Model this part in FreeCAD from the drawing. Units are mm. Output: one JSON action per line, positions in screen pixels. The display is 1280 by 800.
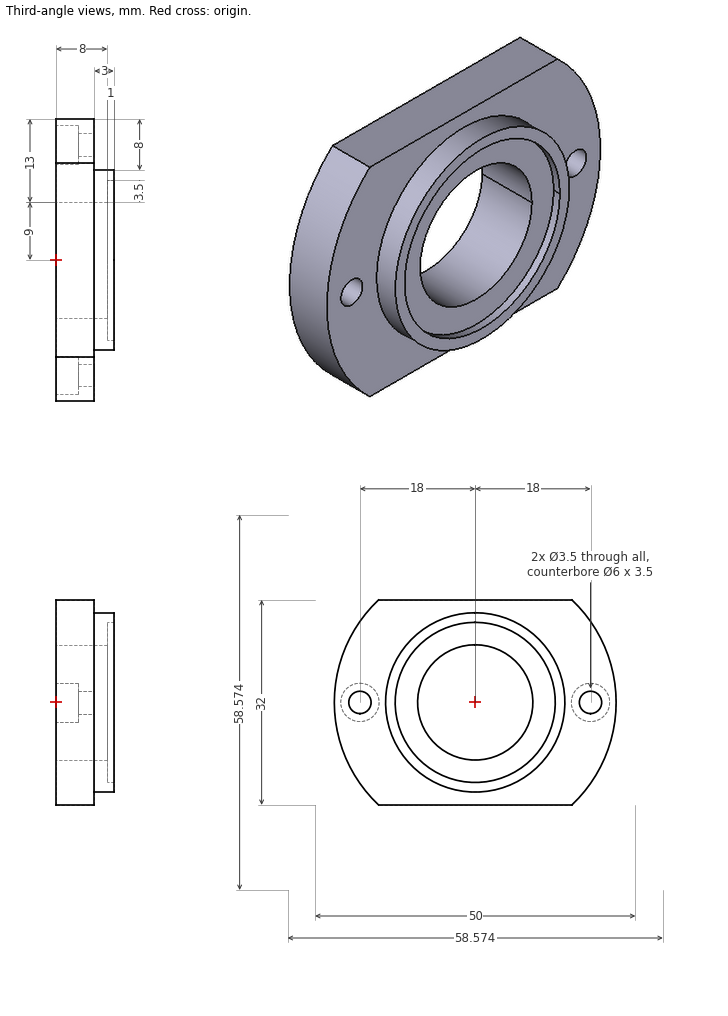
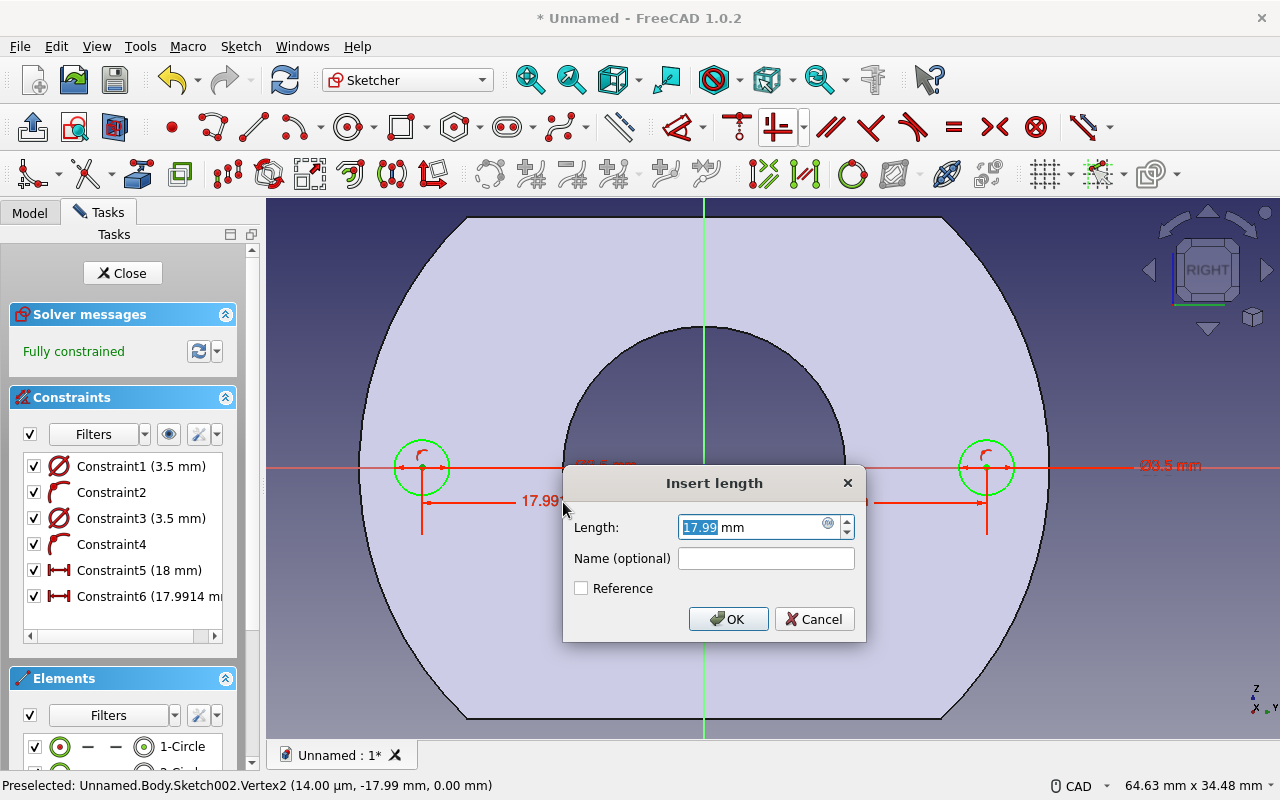
{"action": "type", "text": "18"}
{"action": "key", "text": "Return"}
{"action": "key", "text": "Escape"}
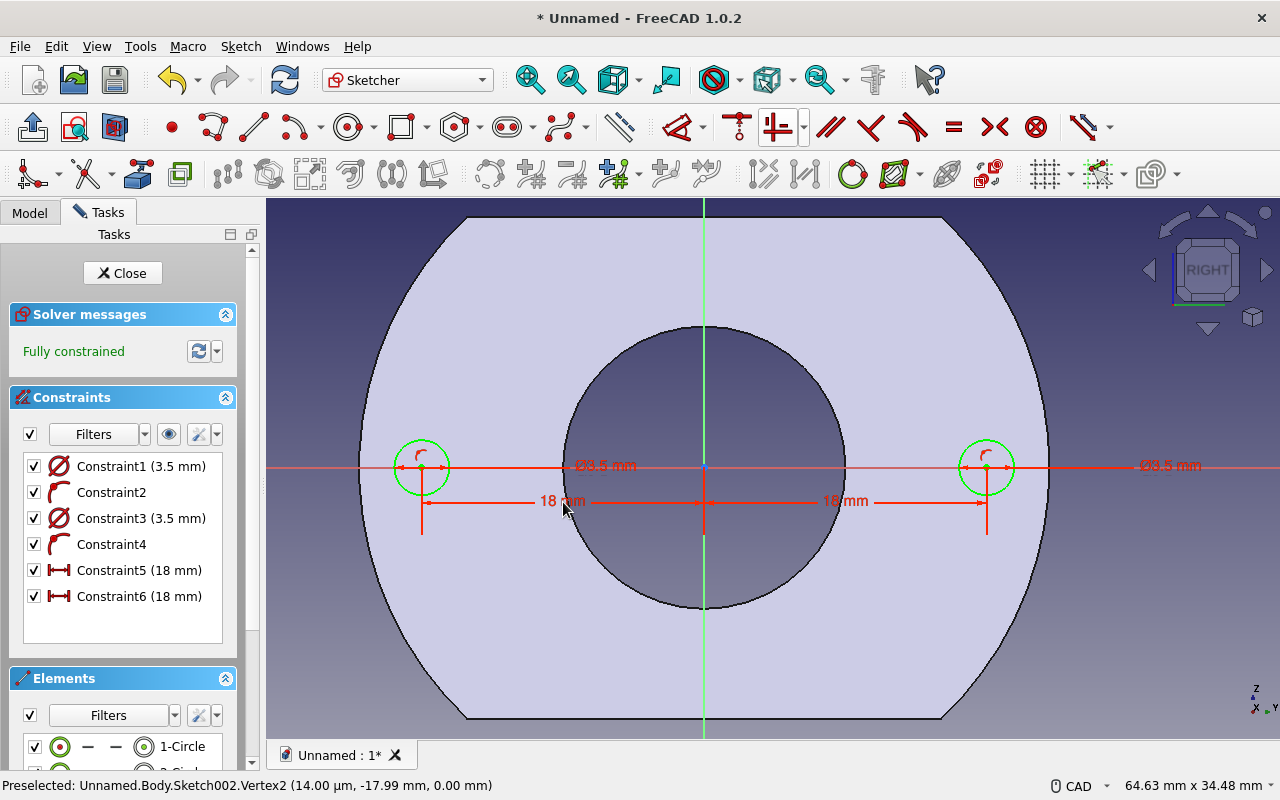
{"action": "left_click", "coordinate": [123, 273]}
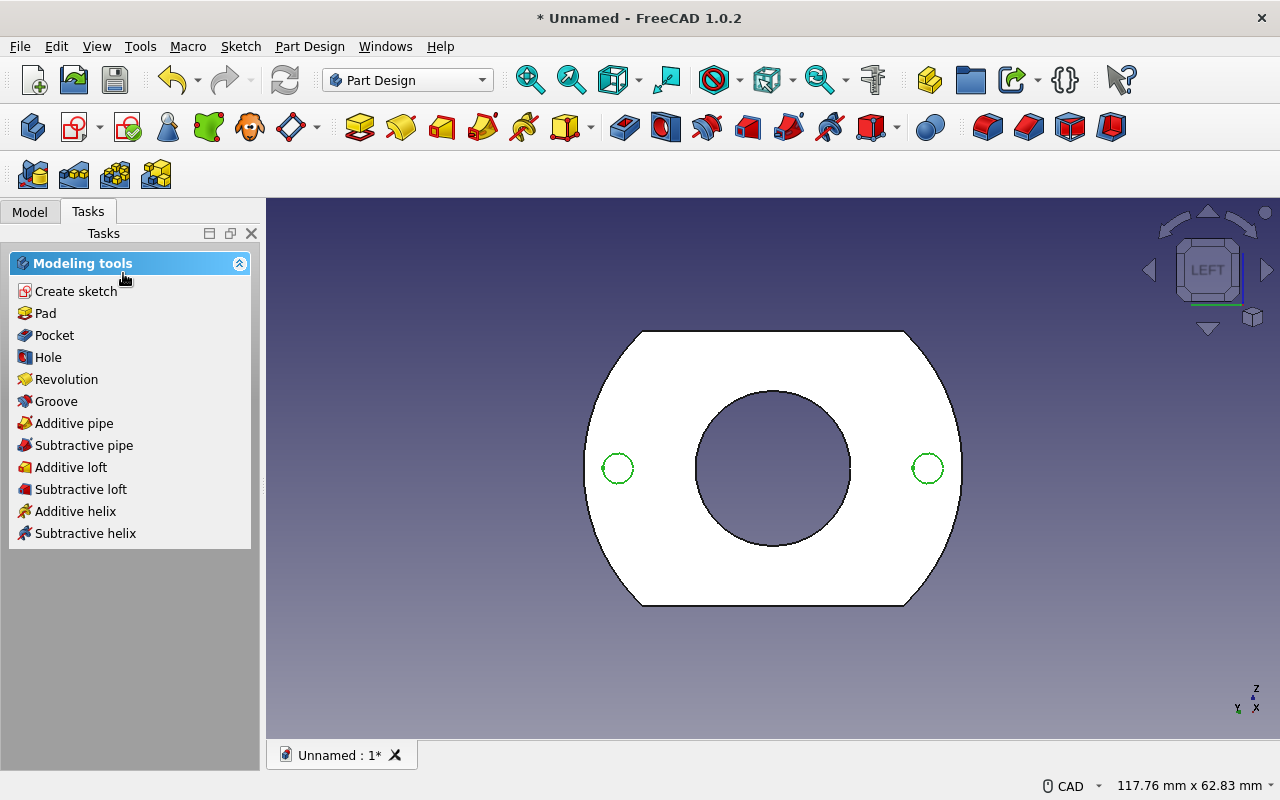
{"action": "left_click", "coordinate": [666, 128]}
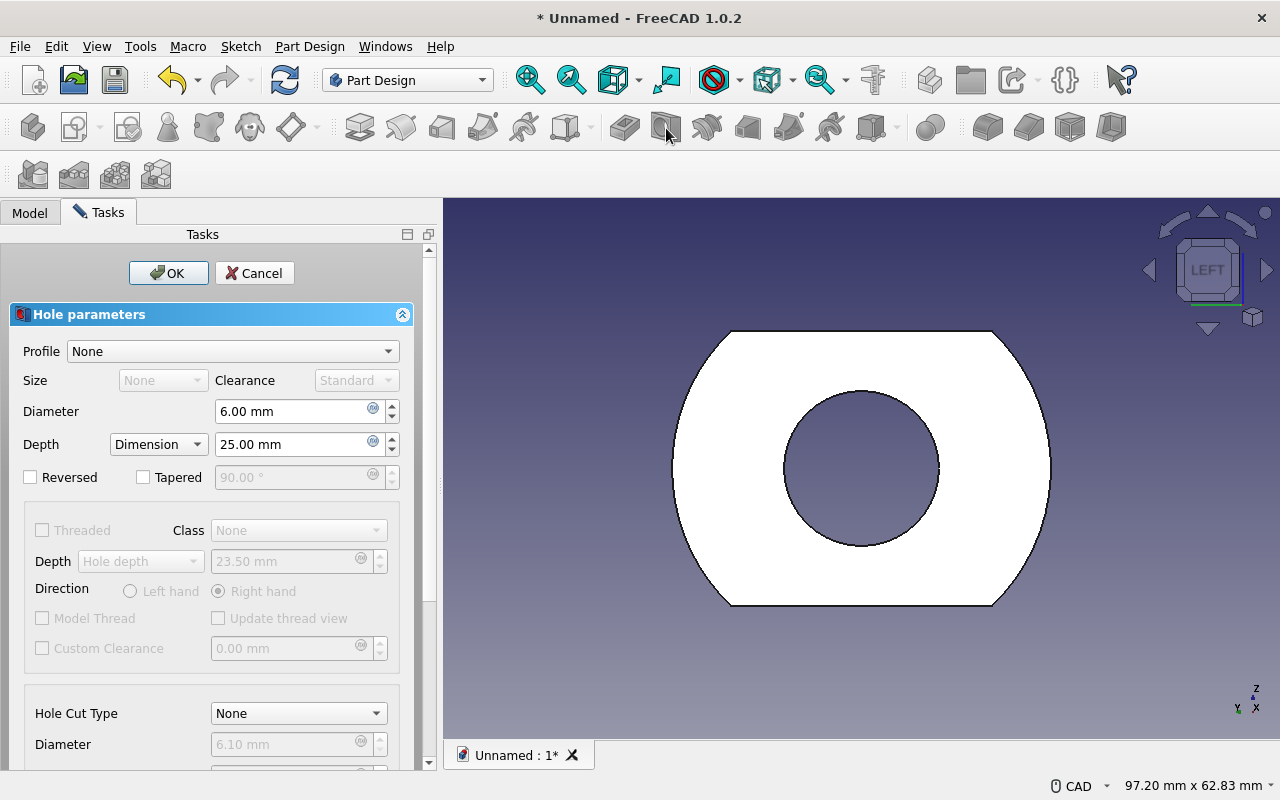
{"action": "triple_click", "coordinate": [300, 412]}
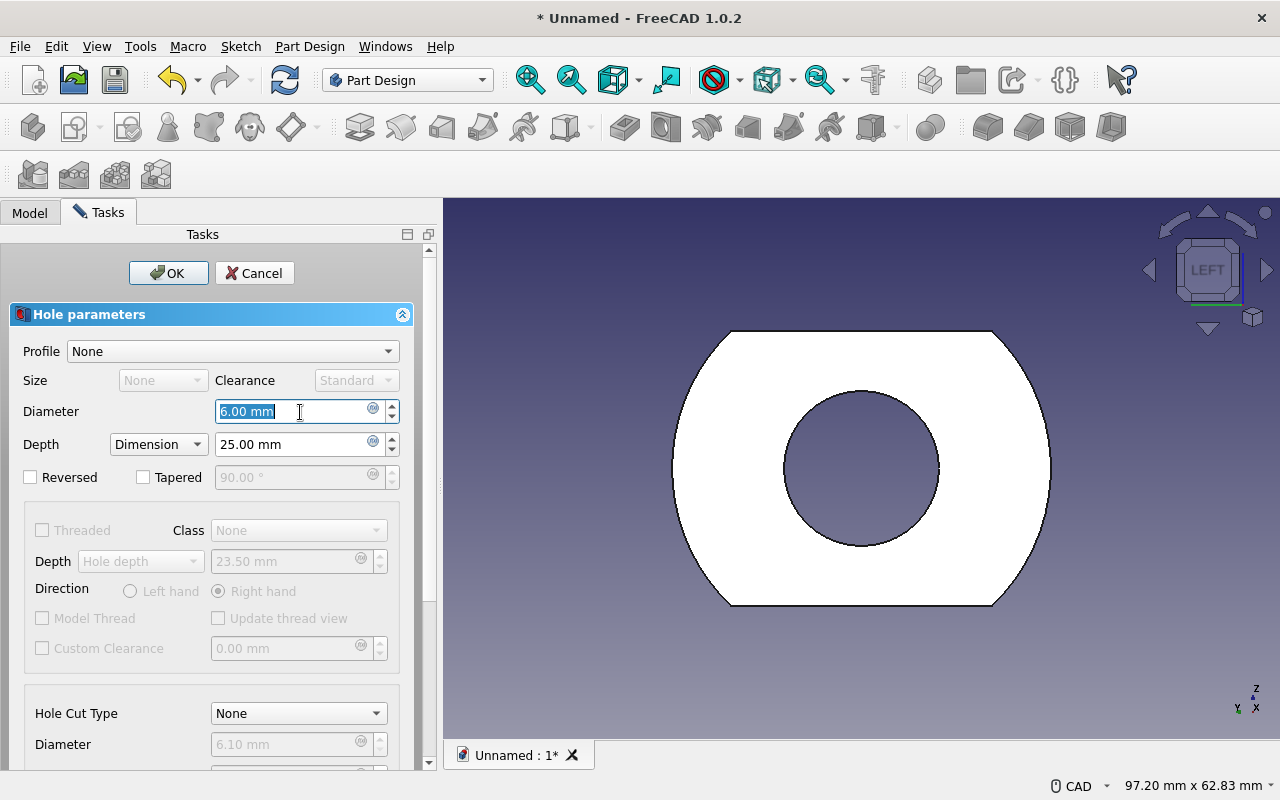
{"action": "type", "text": "3.5"}
{"action": "key", "text": "Tab"}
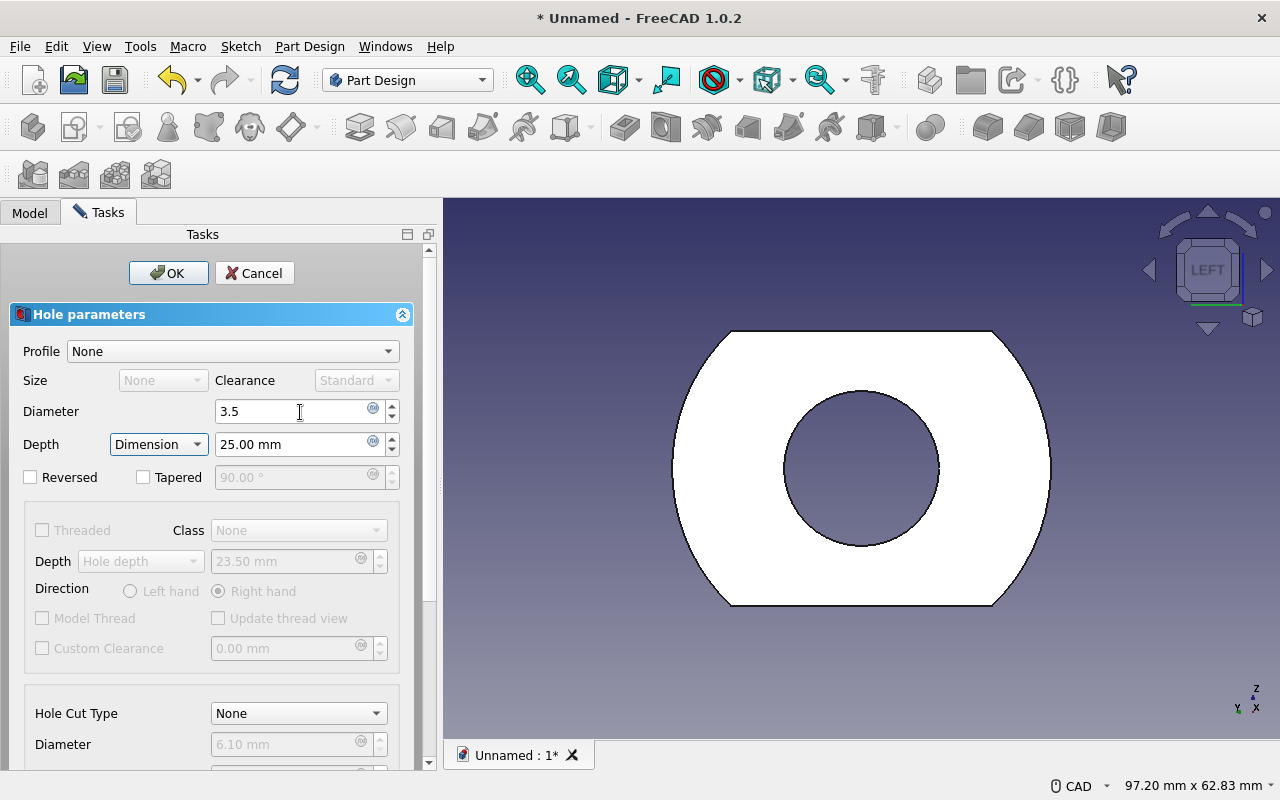
{"action": "left_click", "coordinate": [160, 444]}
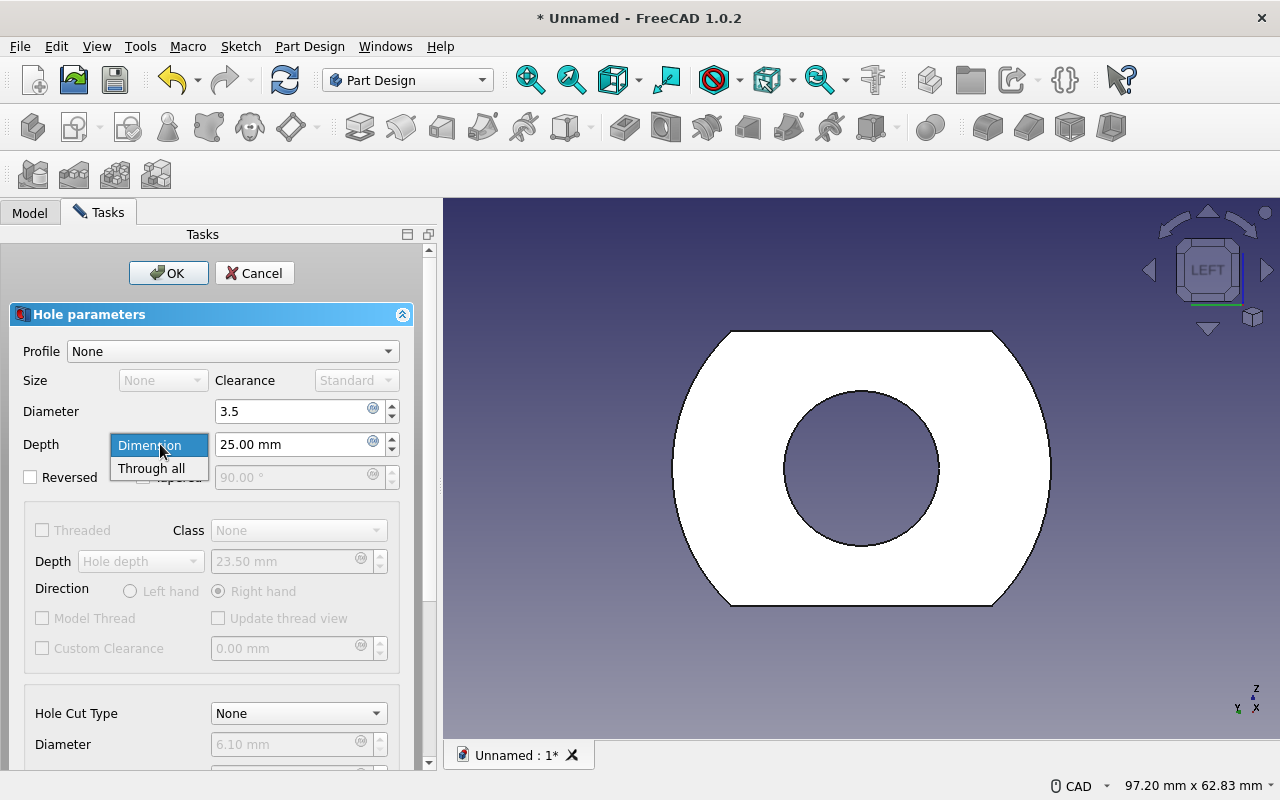
{"action": "left_click", "coordinate": [158, 468]}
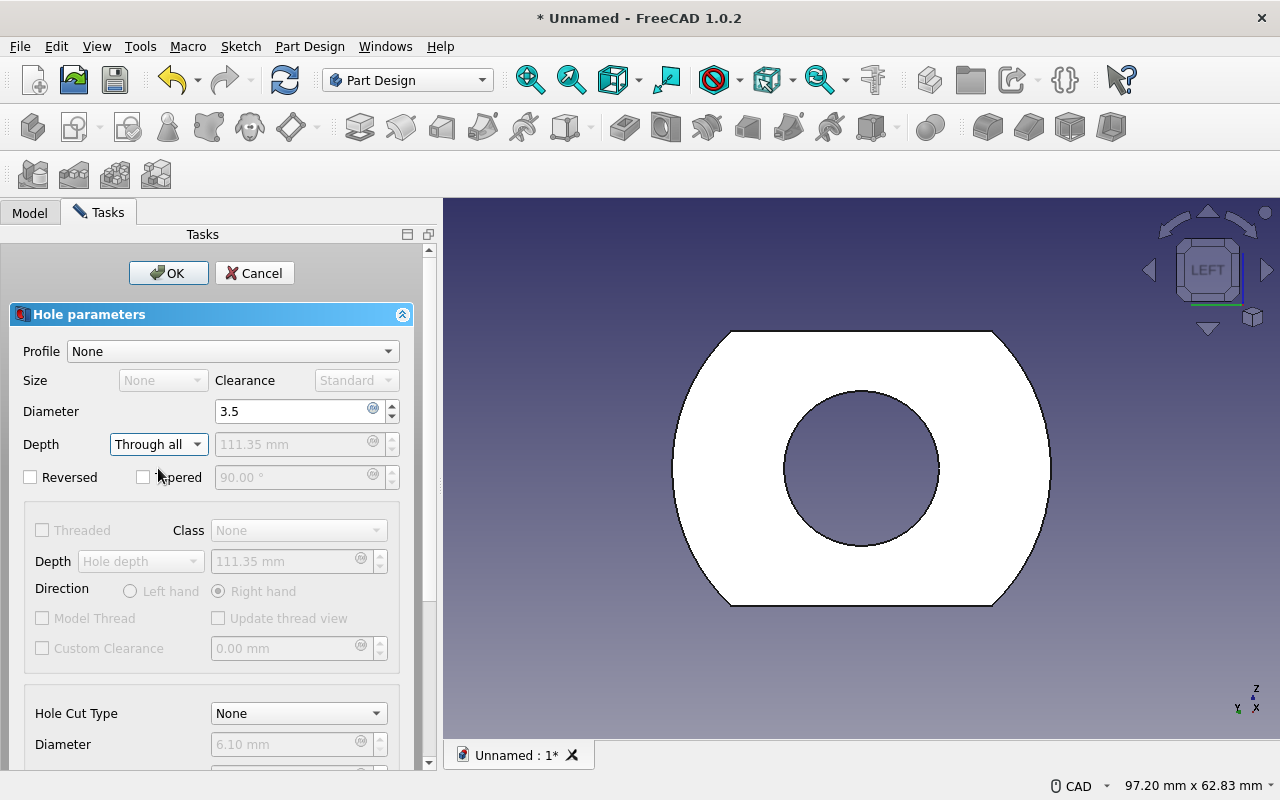
{"action": "left_click", "coordinate": [31, 477]}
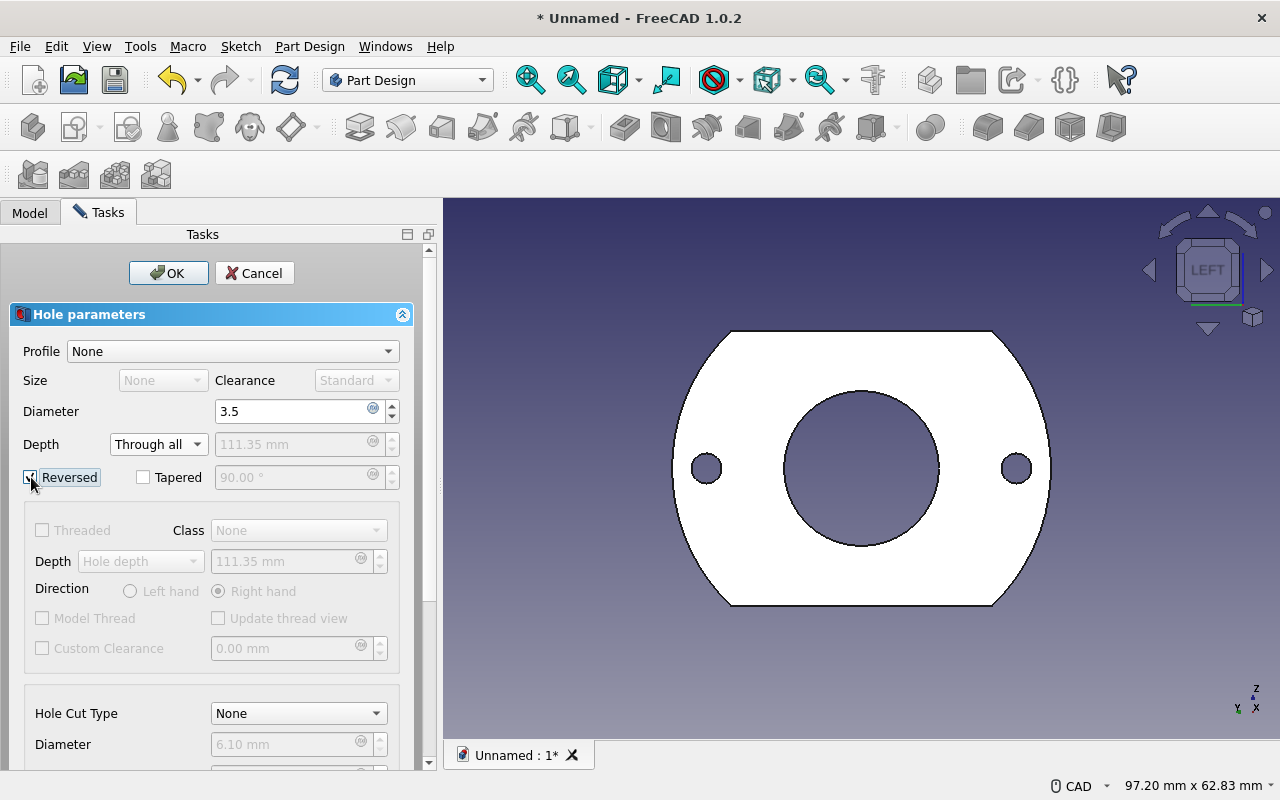
{"action": "left_click", "coordinate": [300, 714]}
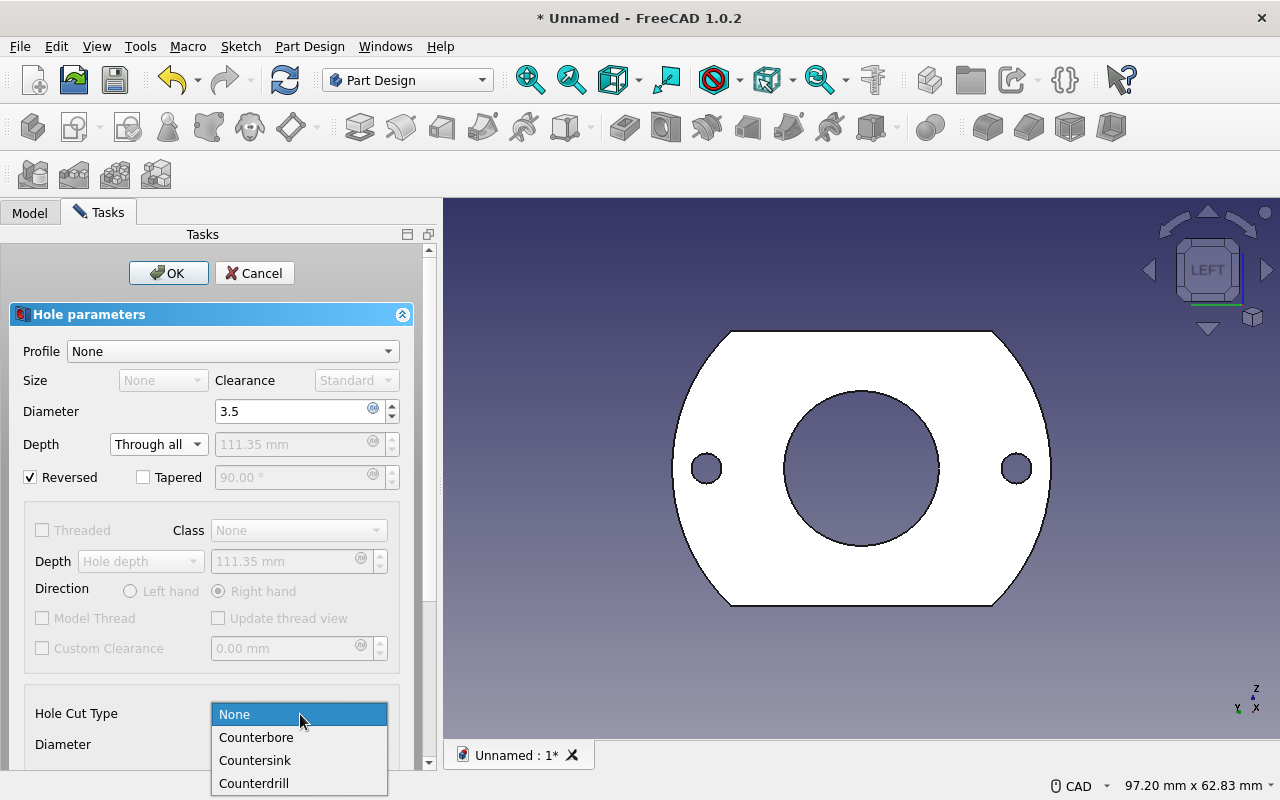
{"action": "left_click", "coordinate": [298, 738]}